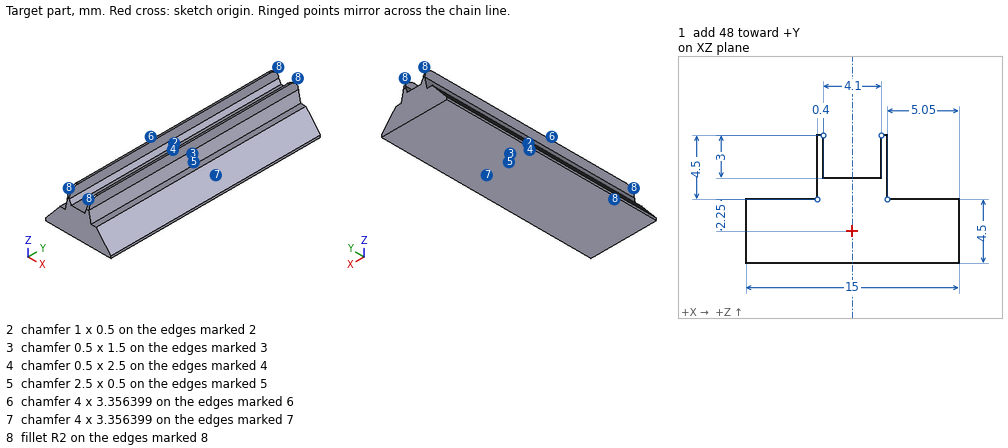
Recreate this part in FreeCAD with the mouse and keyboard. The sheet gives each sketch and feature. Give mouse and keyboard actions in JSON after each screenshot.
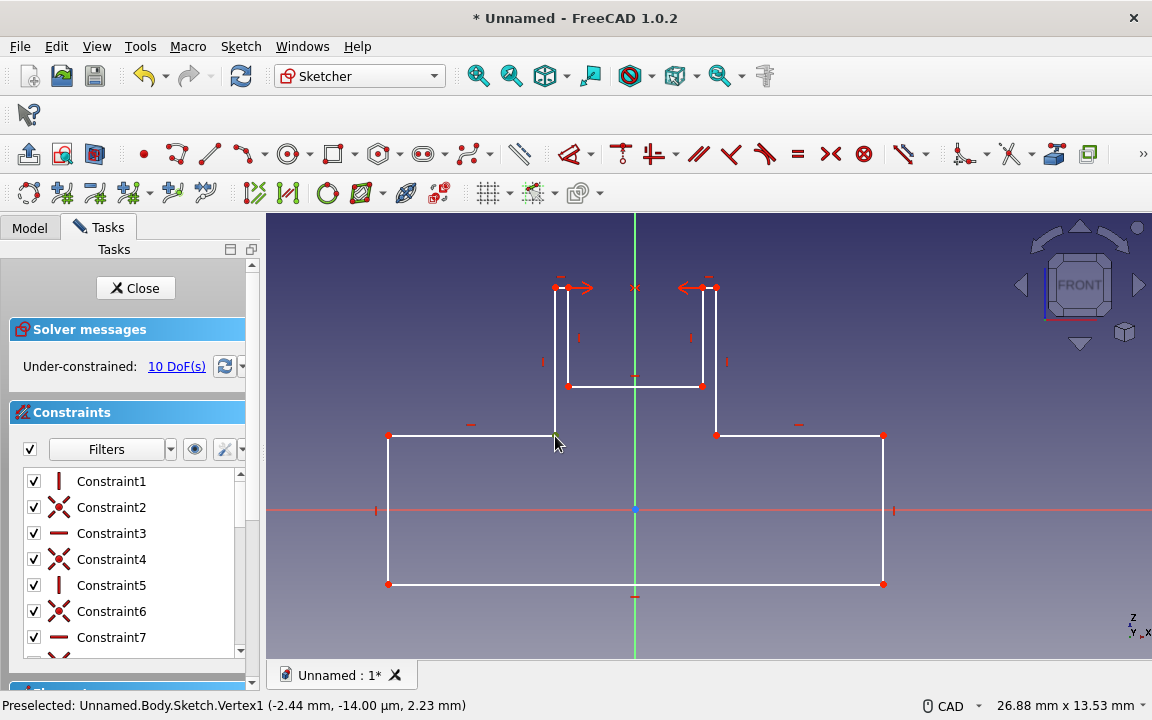
{"action": "left_click", "coordinate": [716, 436]}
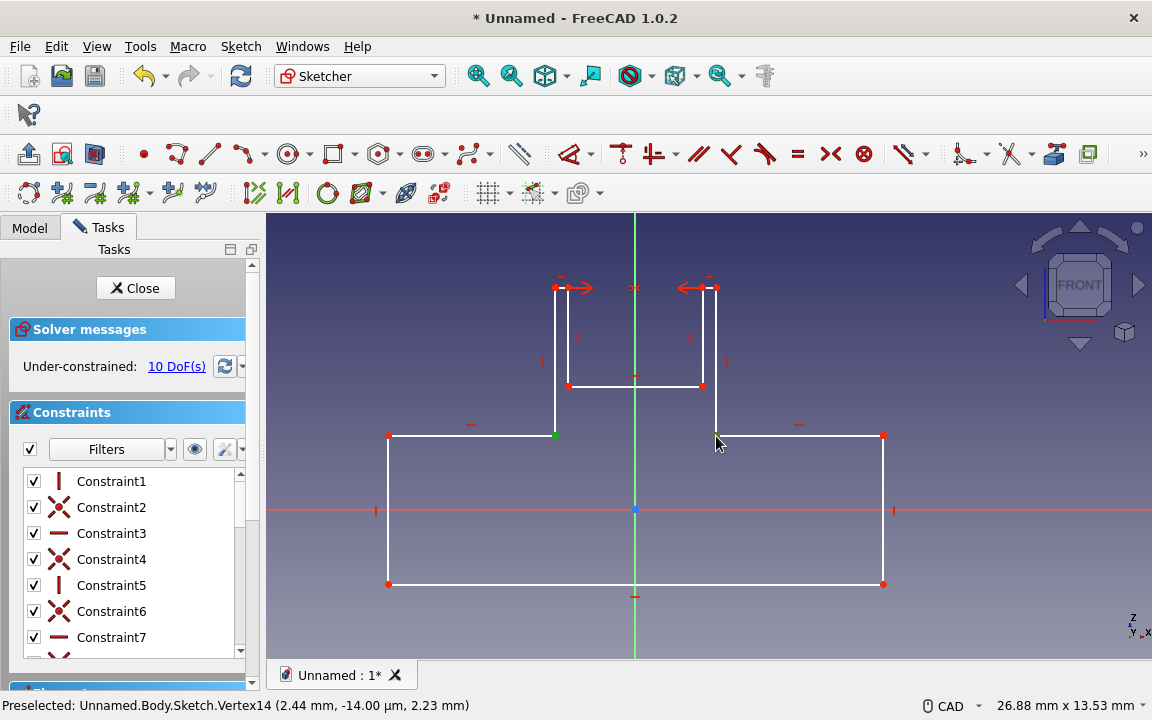
{"action": "left_click", "coordinate": [635, 547]}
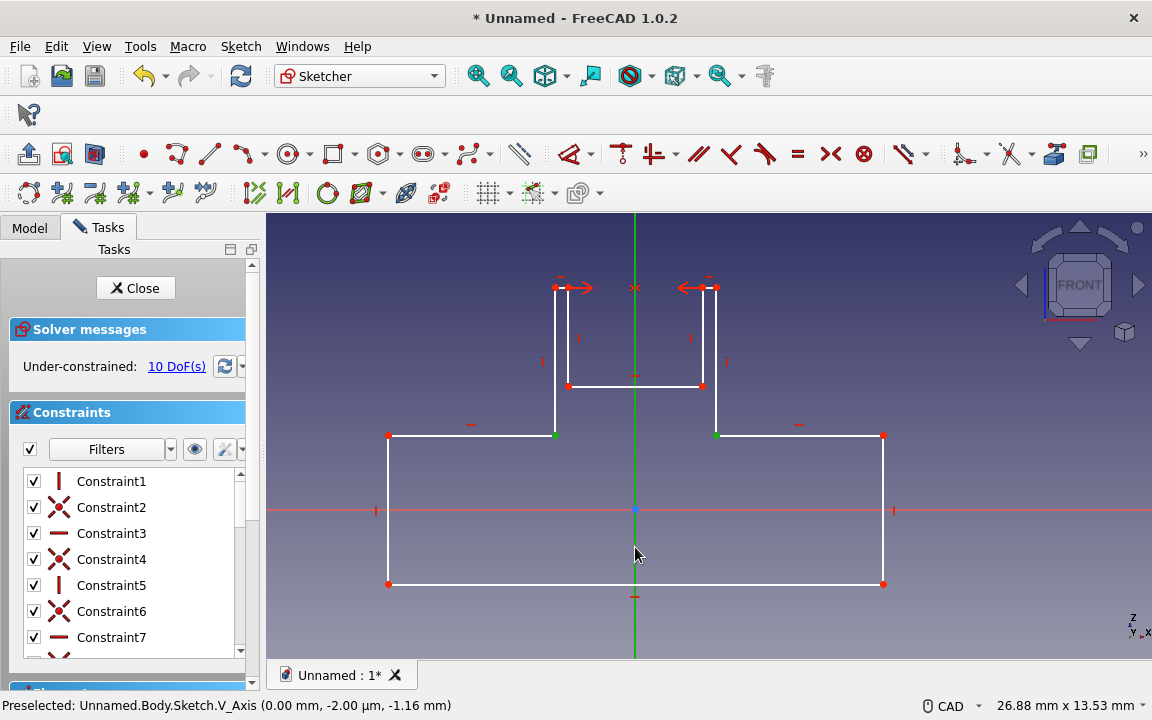
{"action": "left_click", "coordinate": [831, 154]}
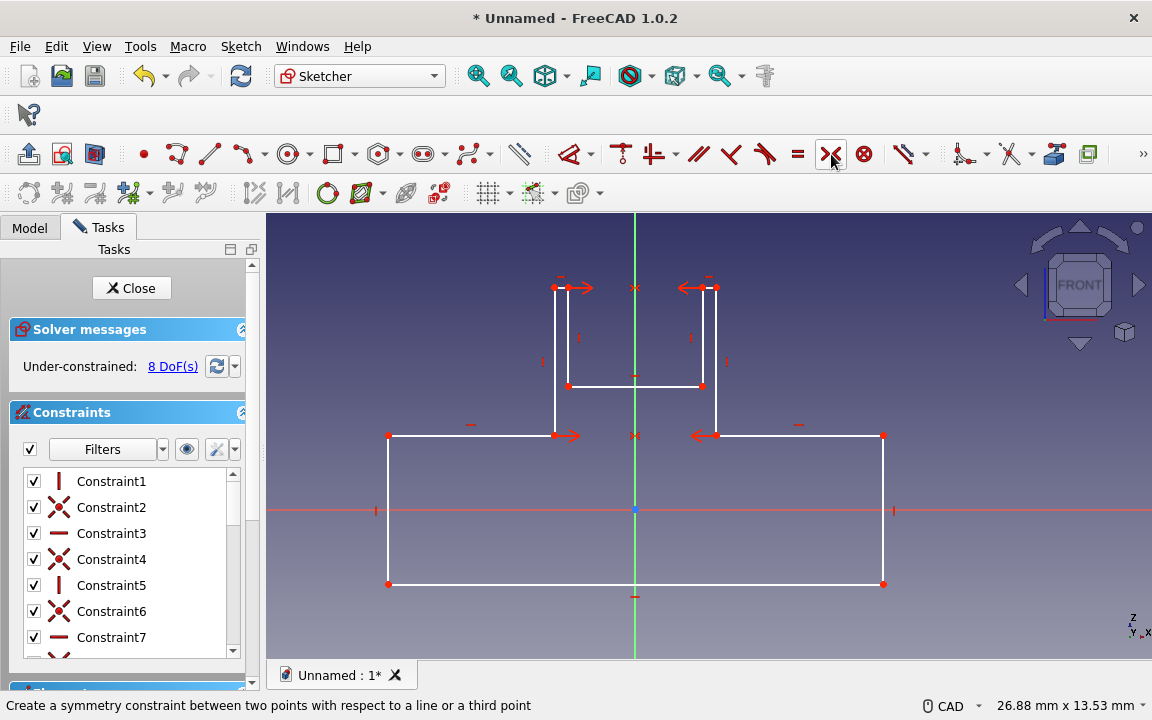
{"action": "left_click", "coordinate": [568, 154]}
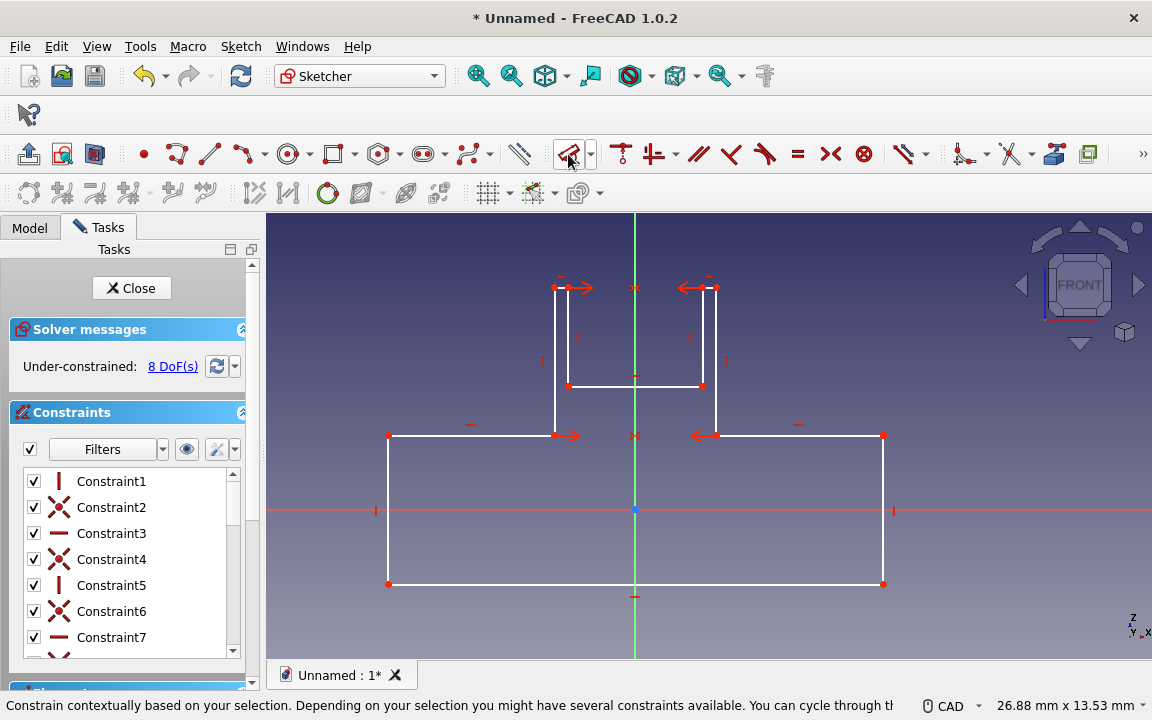
{"action": "left_click", "coordinate": [568, 318]}
{"action": "left_click", "coordinate": [534, 337]}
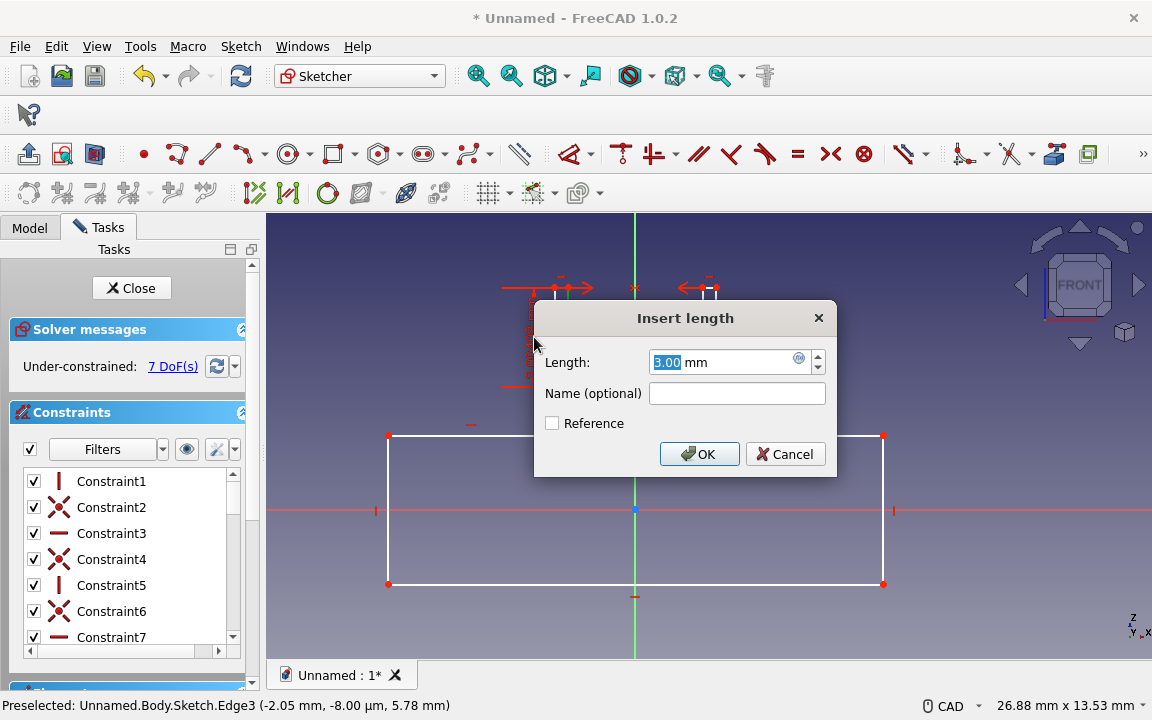
{"action": "type", "text": "3"}
{"action": "key", "text": "Return"}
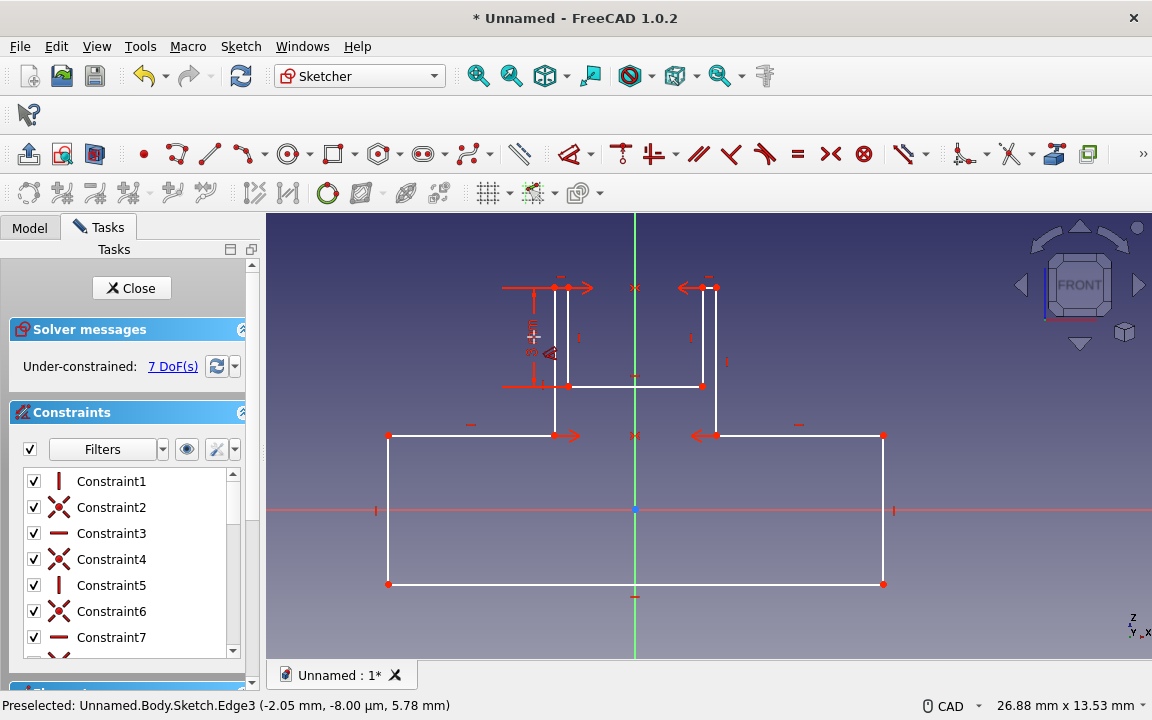
{"action": "left_click", "coordinate": [734, 585]}
{"action": "left_click", "coordinate": [522, 619]}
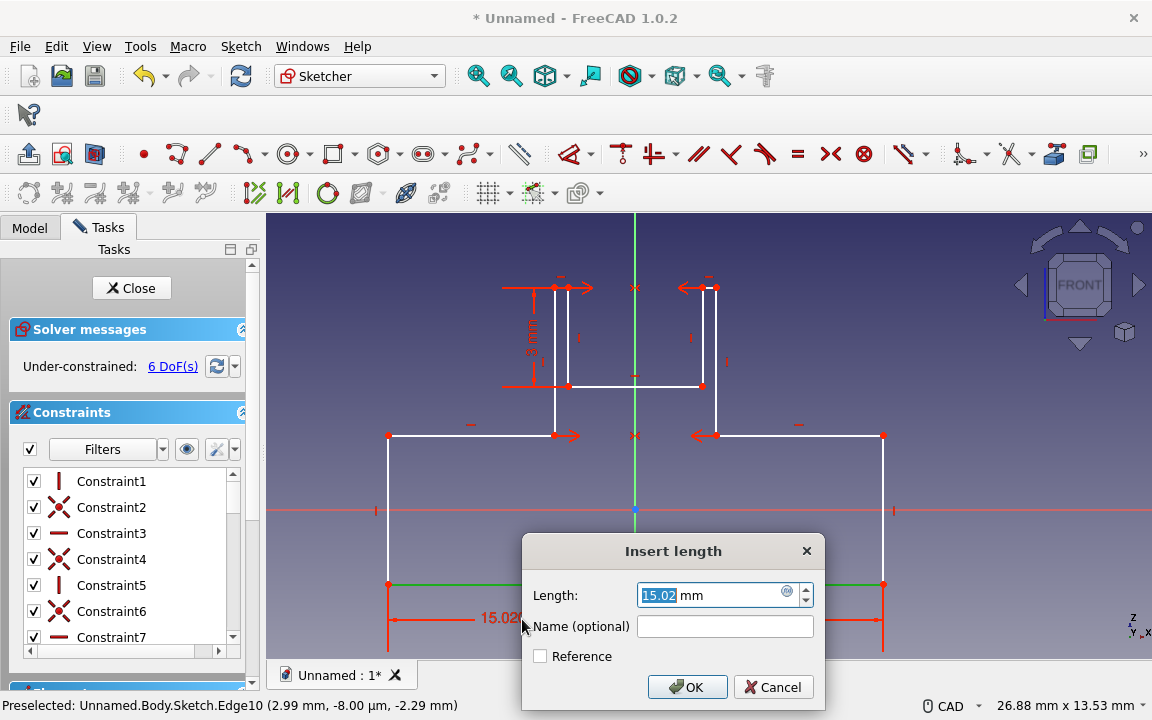
{"action": "type", "text": "15"}
{"action": "key", "text": "Return"}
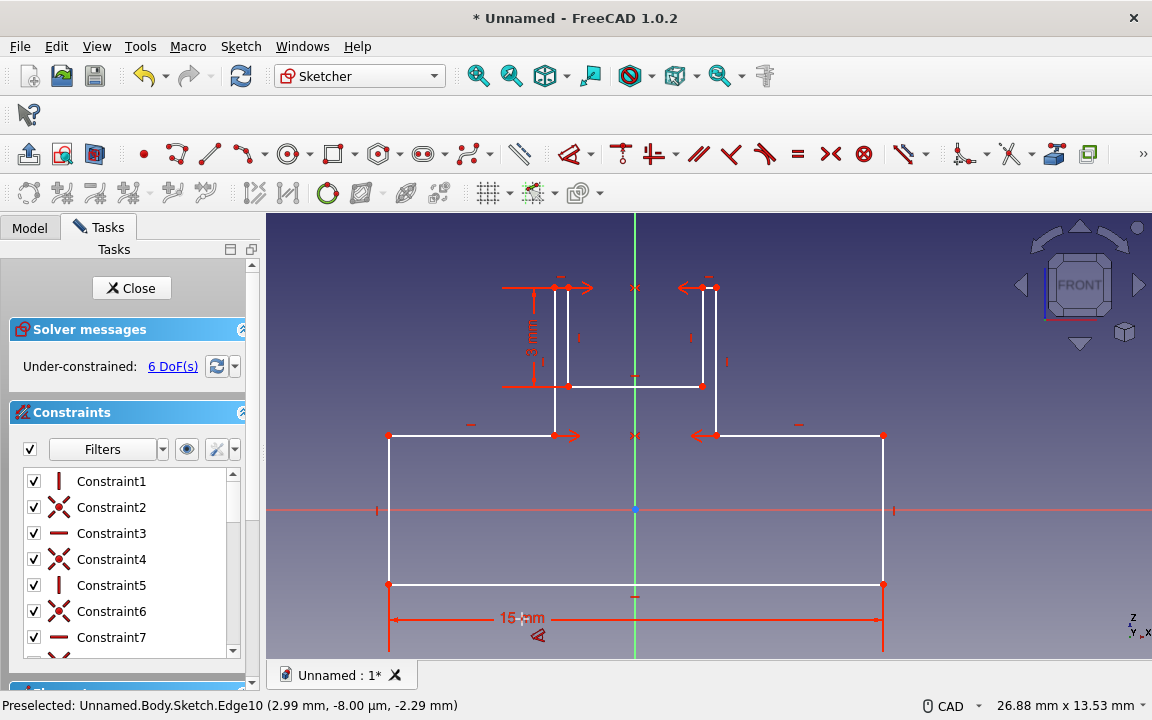
{"action": "left_click", "coordinate": [555, 392]}
{"action": "left_click", "coordinate": [521, 362]}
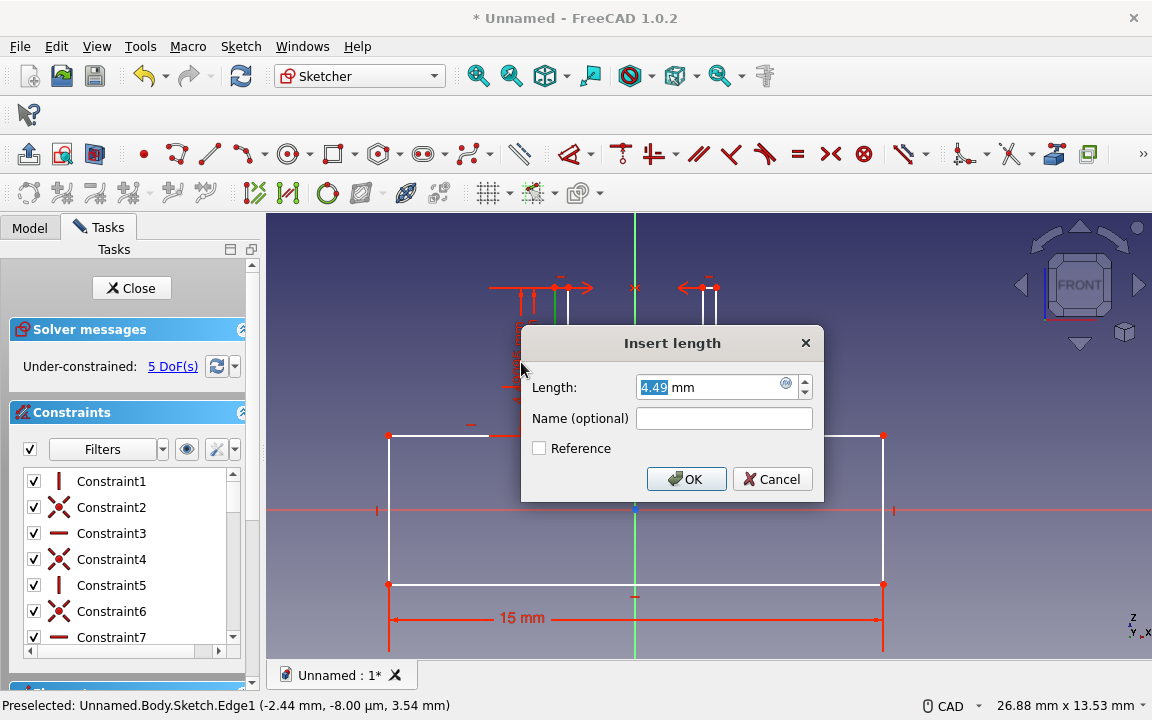
{"action": "type", "text": "4.5"}
{"action": "key", "text": "Return"}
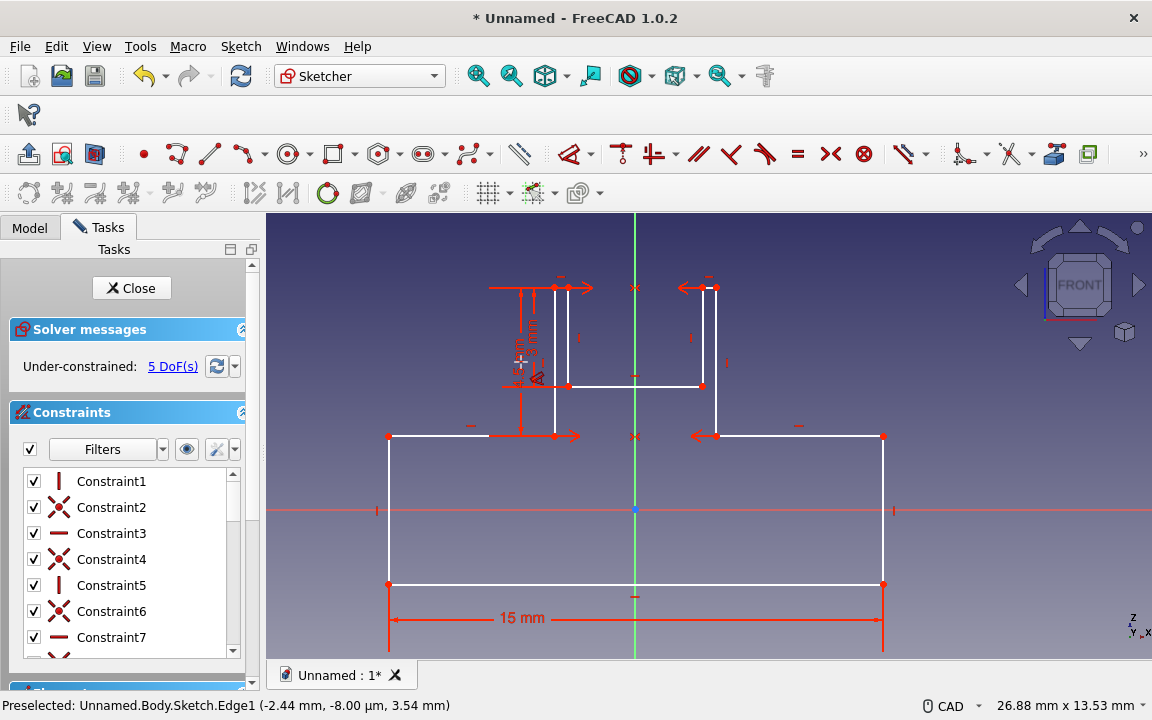
{"action": "scroll", "coordinate": [561, 288], "scroll_direction": "up", "scroll_amount": 6}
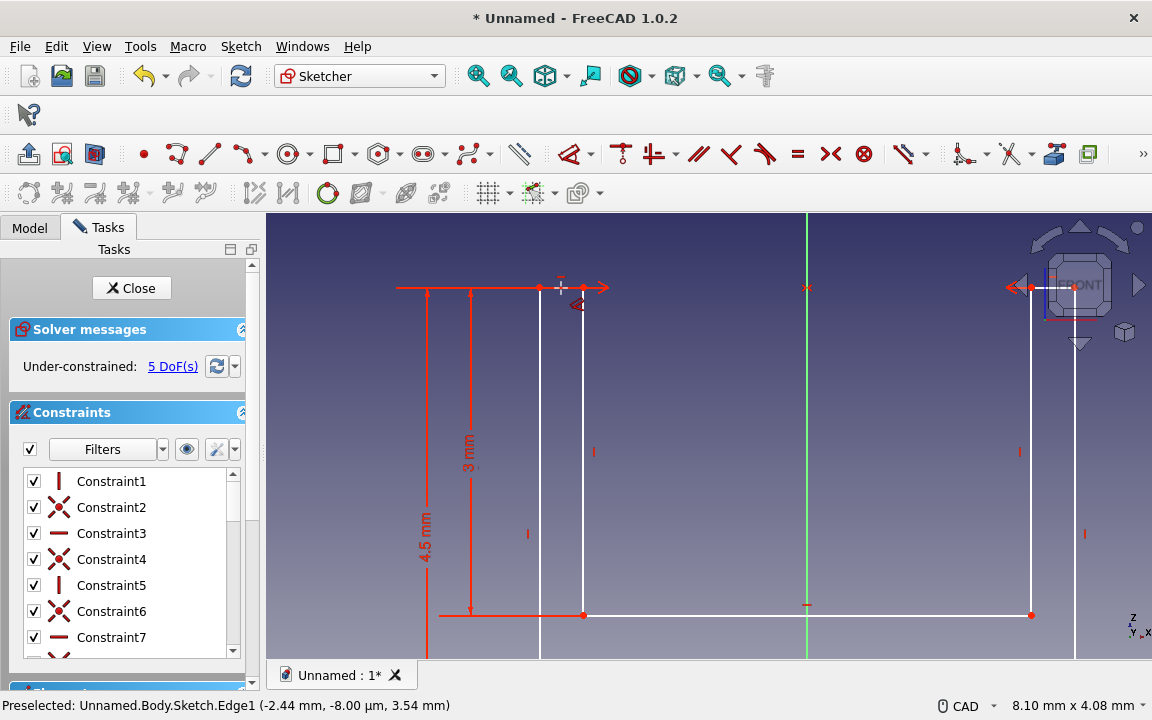
{"action": "left_click", "coordinate": [562, 288]}
{"action": "left_click", "coordinate": [562, 254]}